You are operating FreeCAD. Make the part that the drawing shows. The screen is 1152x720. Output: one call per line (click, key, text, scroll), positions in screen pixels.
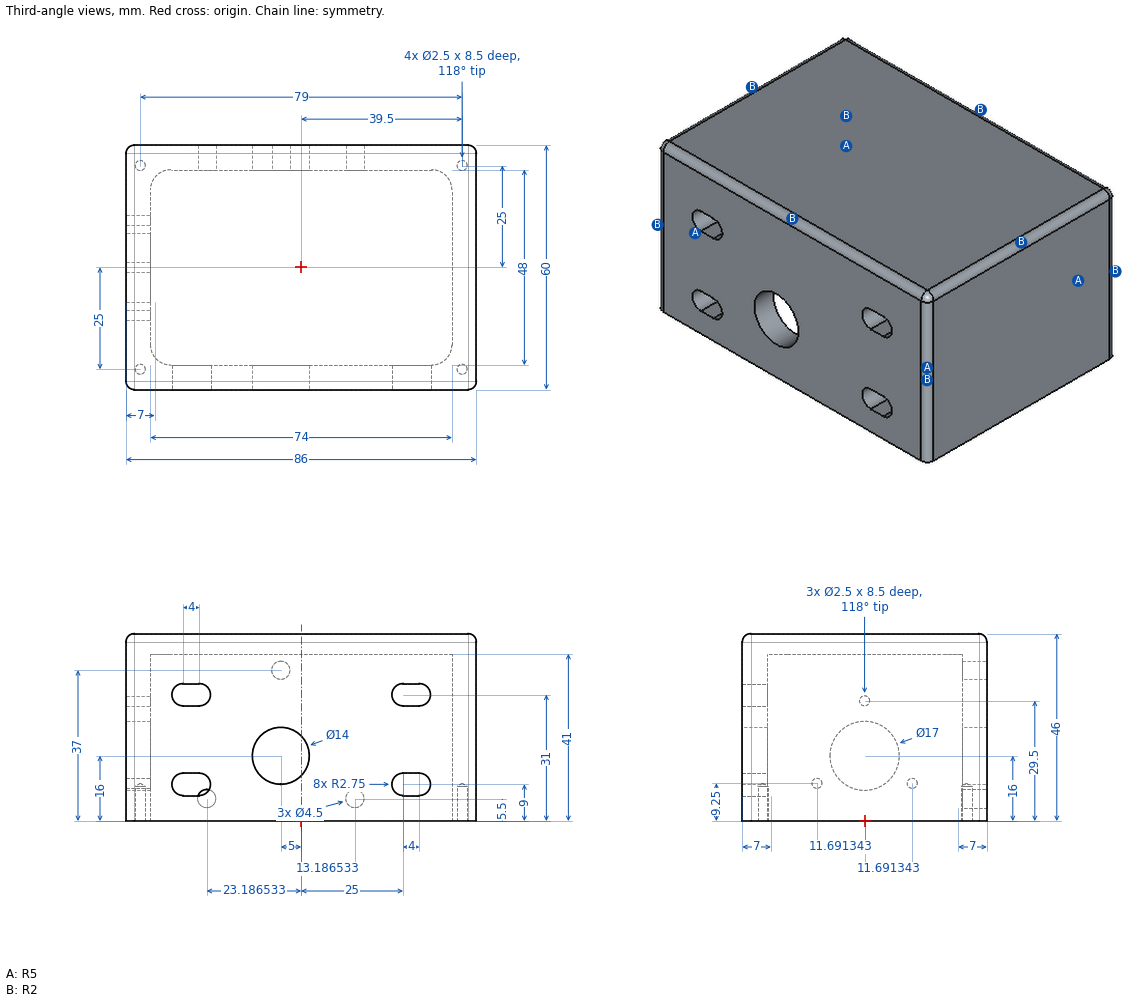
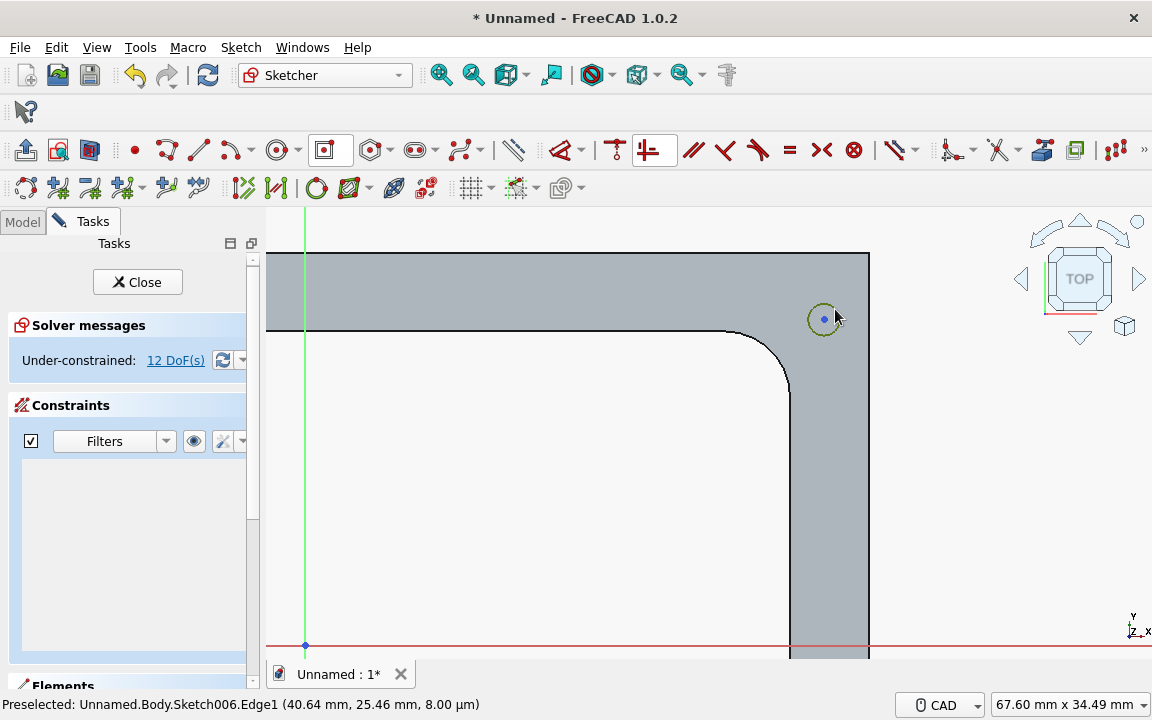
scroll(836, 309, down, 5)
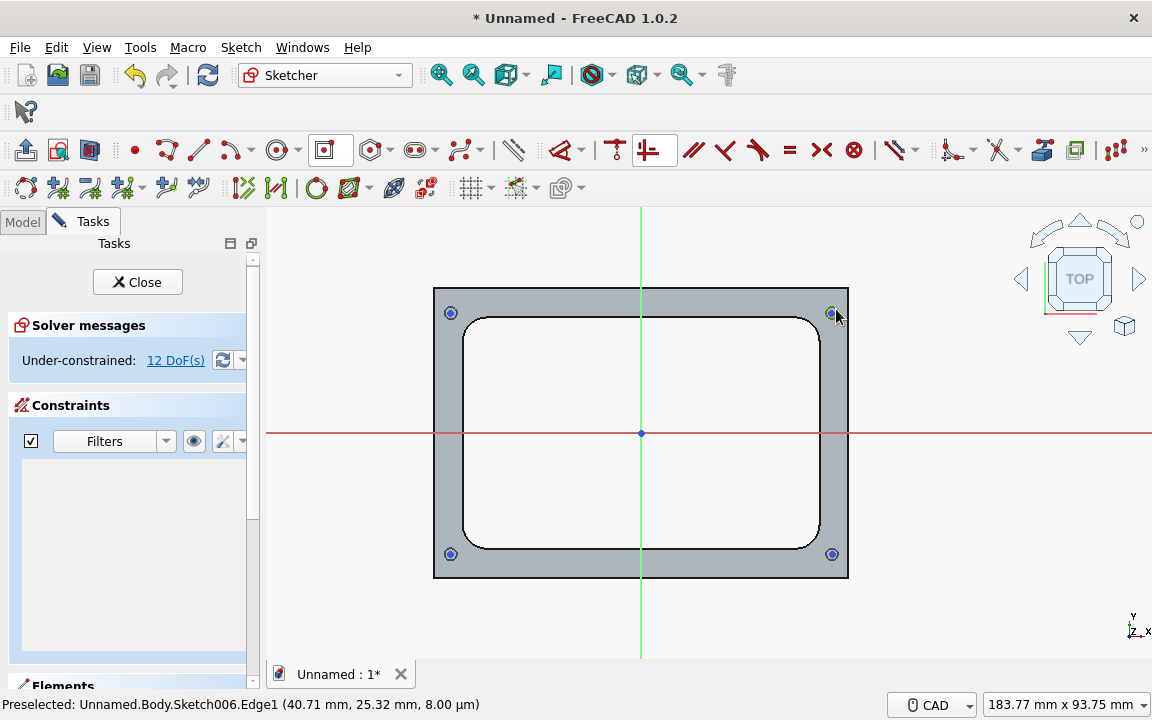
scroll(455, 309, up, 5)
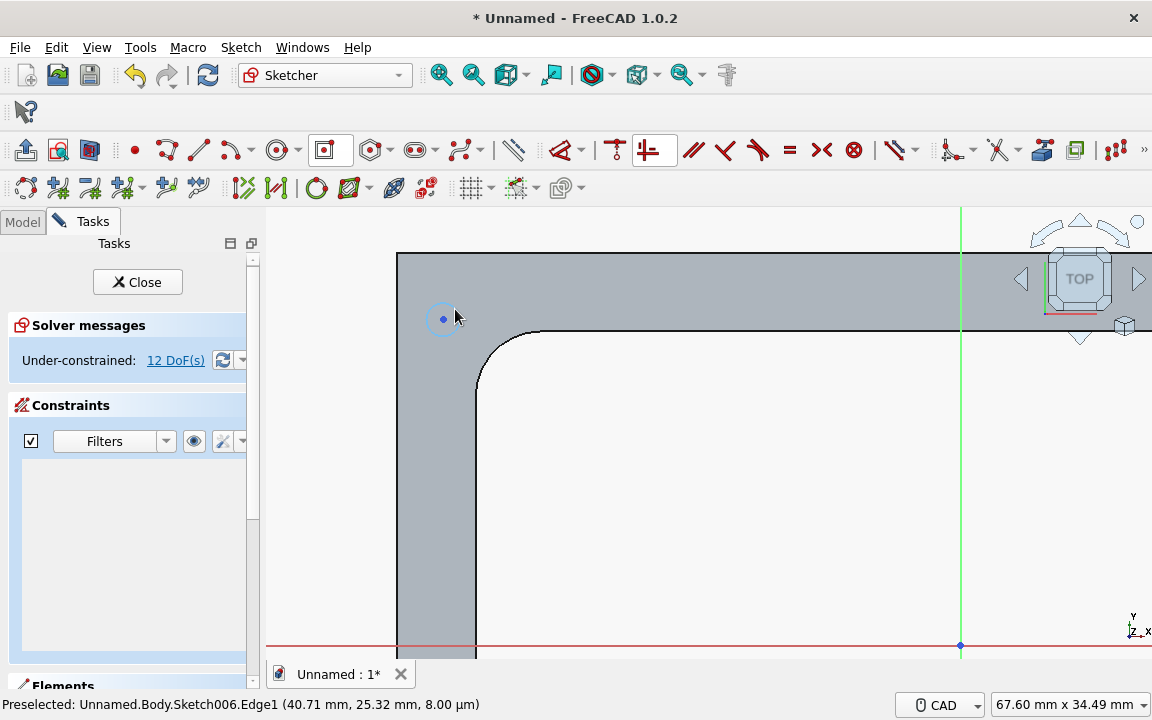
click(455, 308)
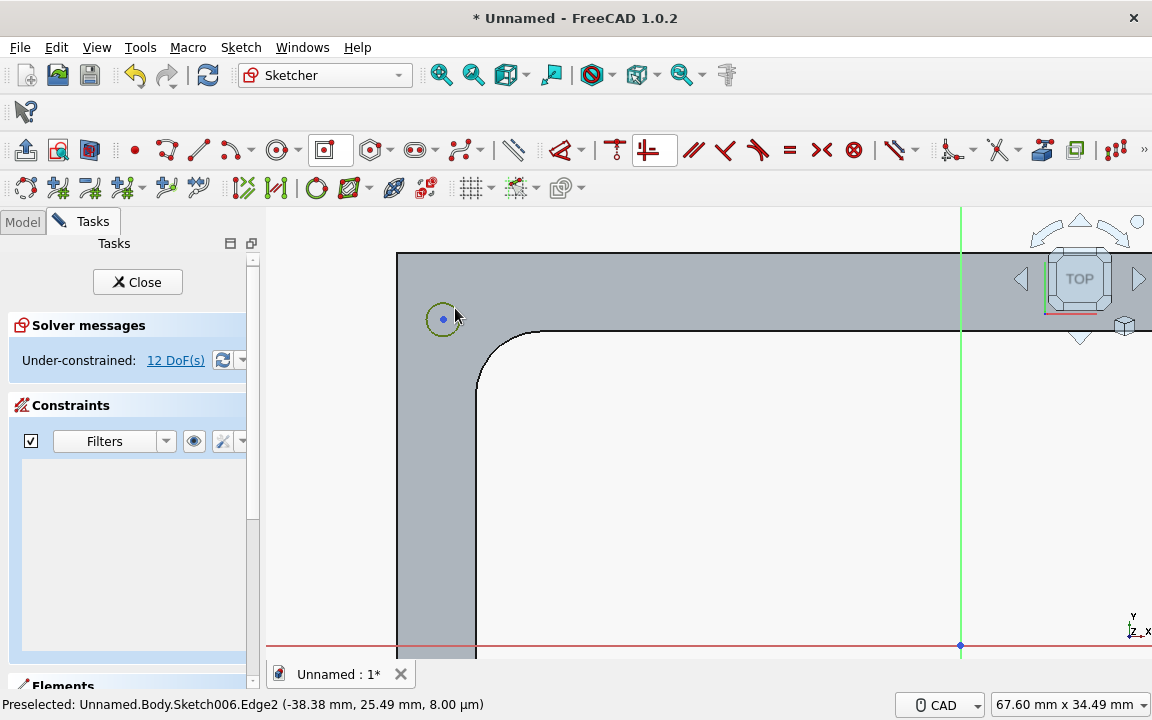
scroll(454, 309, down, 5)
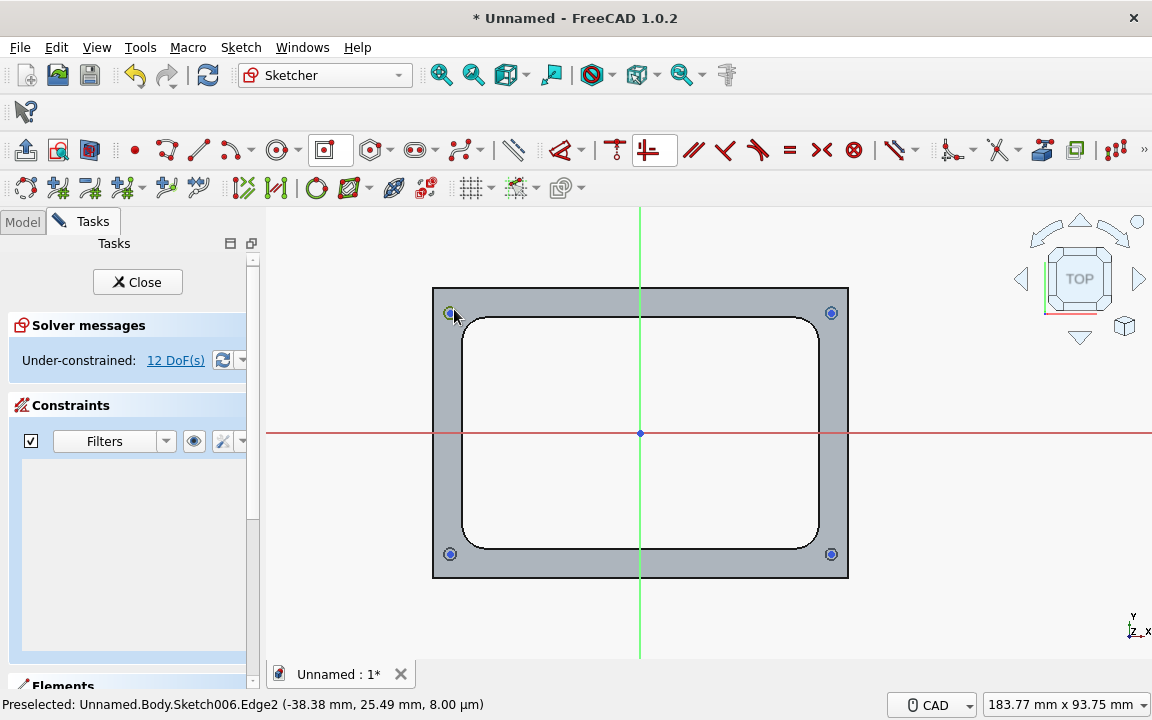
scroll(454, 550, up, 5)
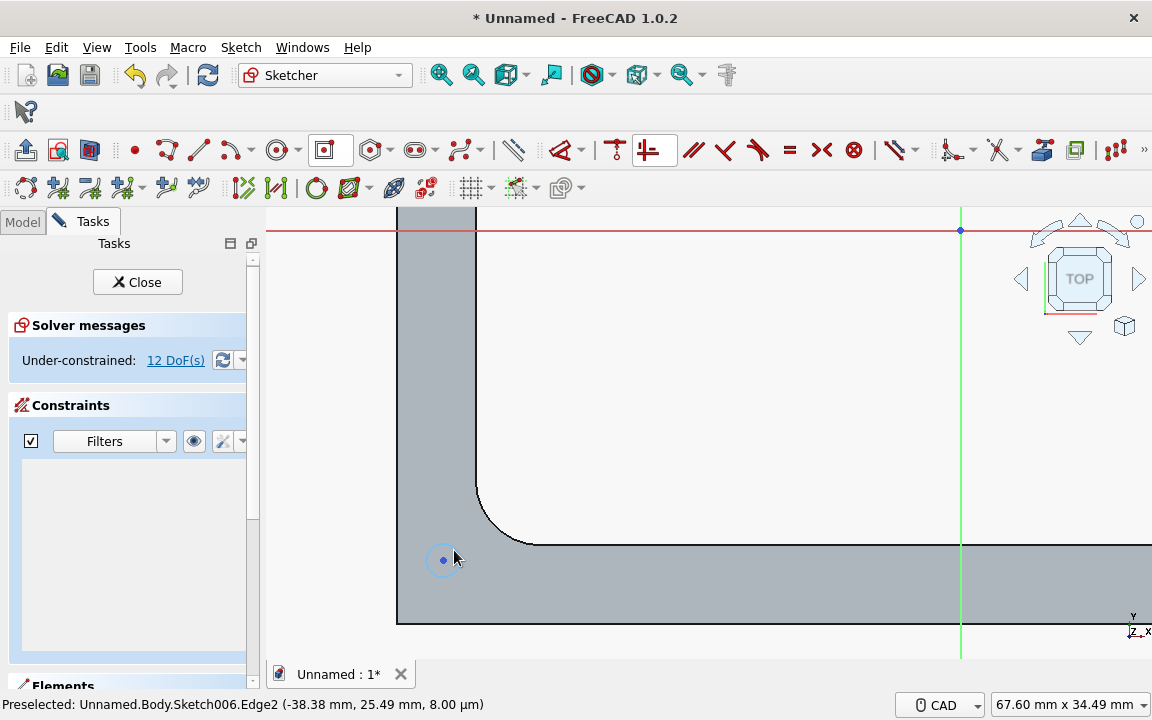
click(455, 549)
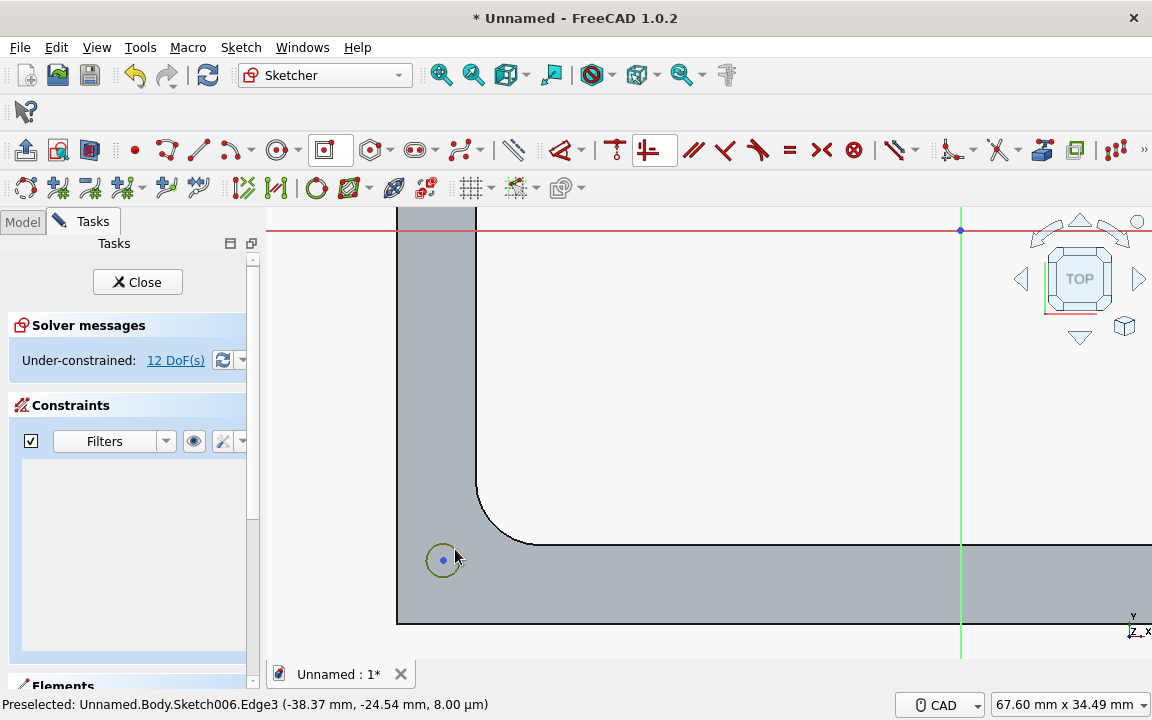
scroll(454, 551, down, 5)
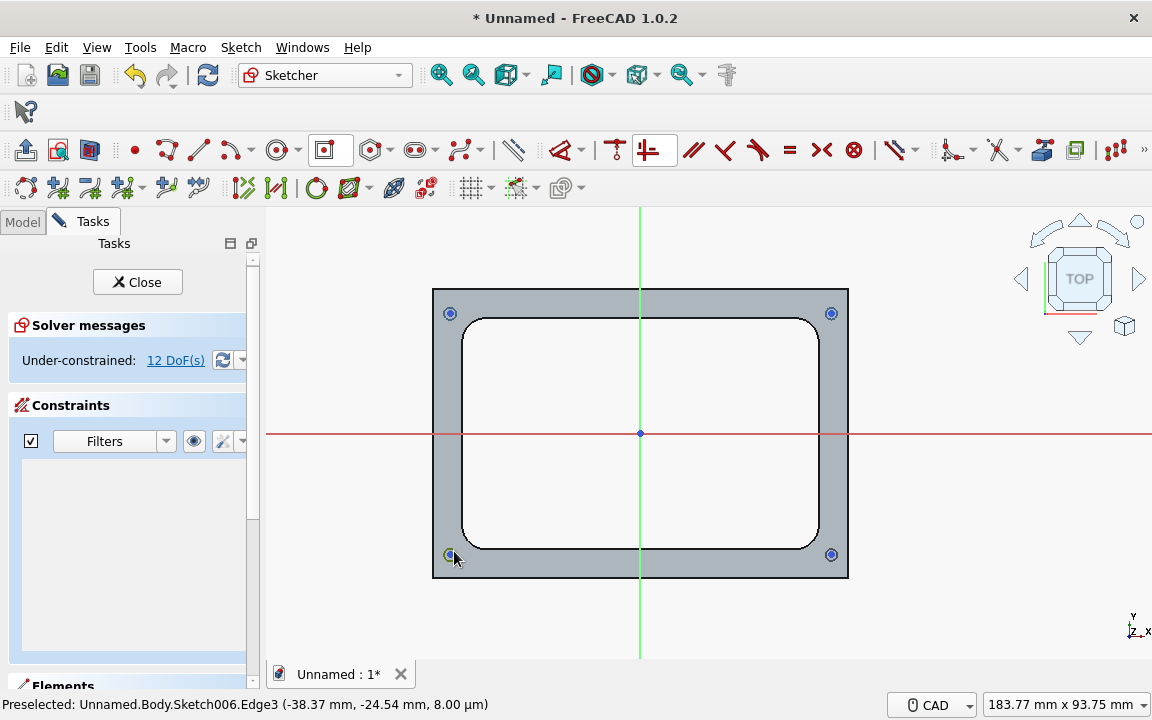
scroll(835, 551, up, 5)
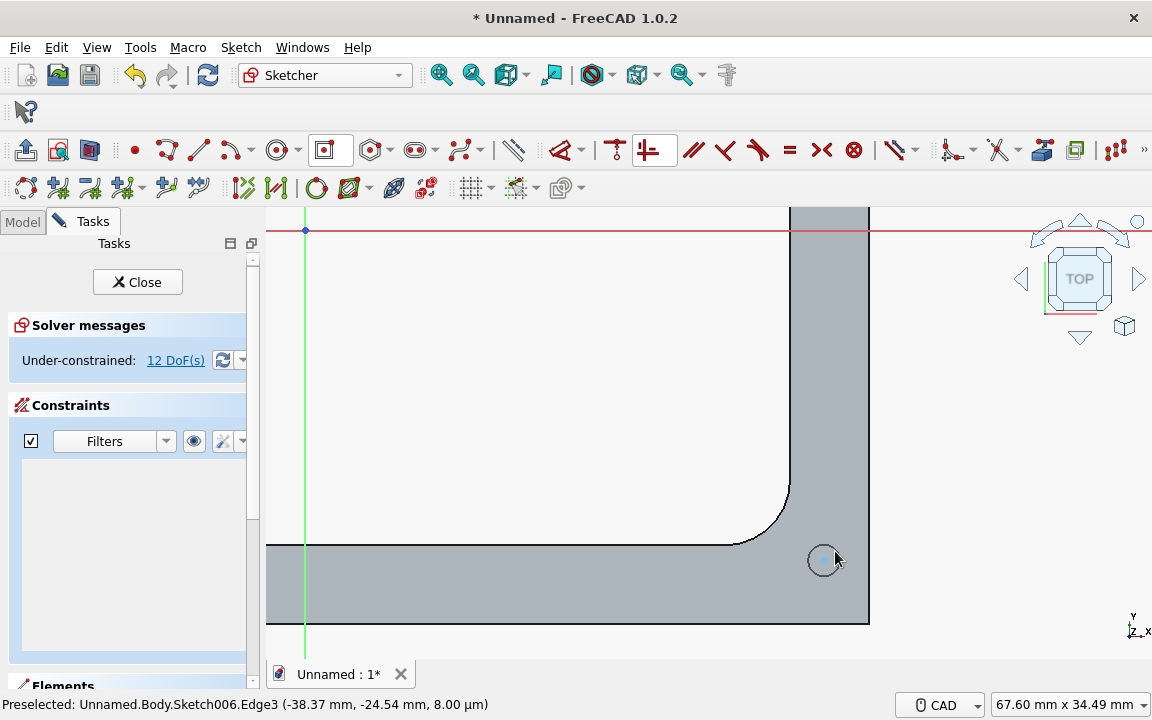
click(835, 549)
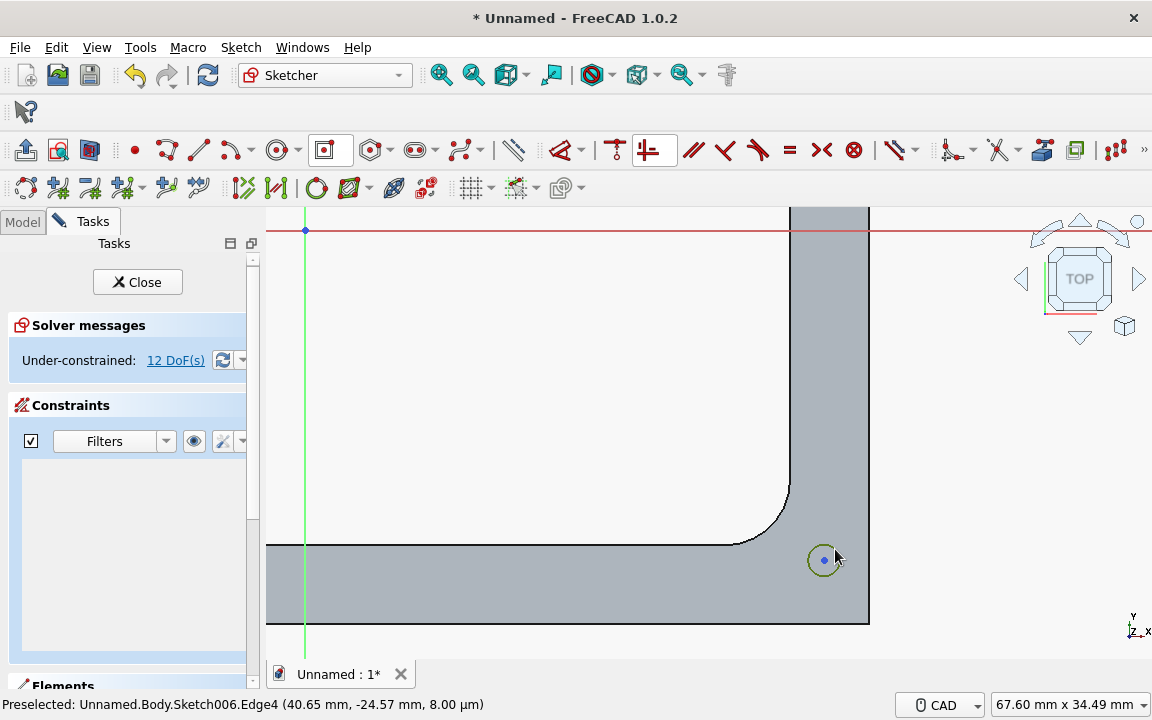
click(790, 150)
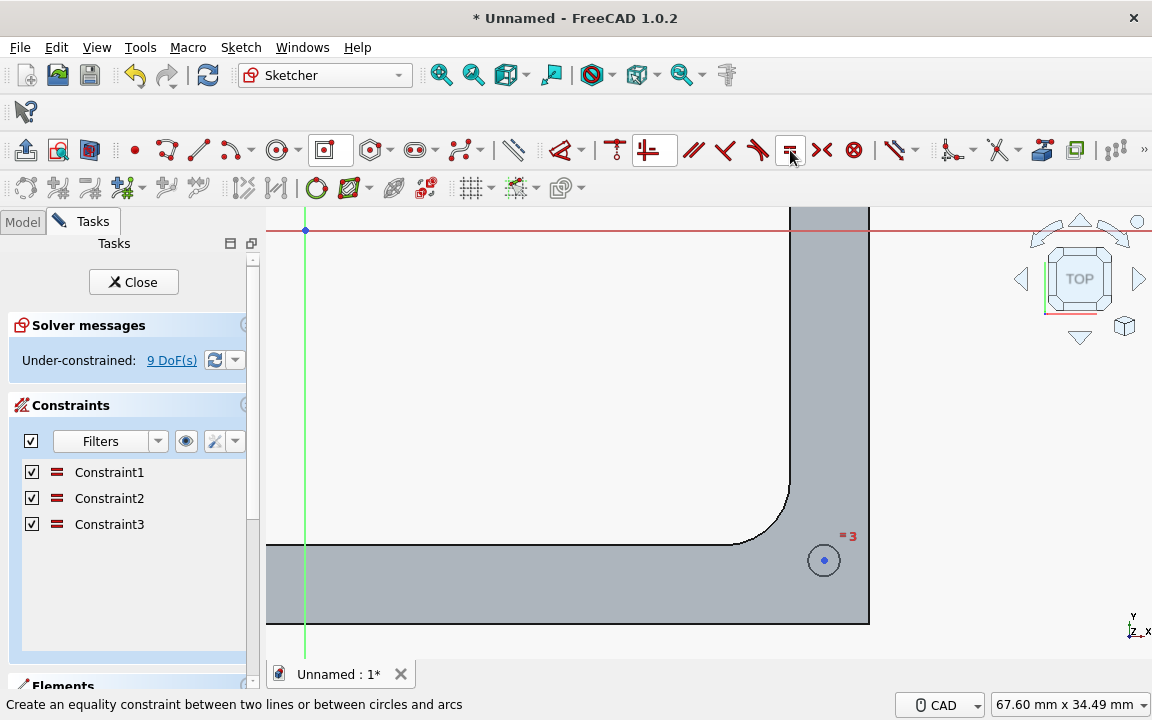
scroll(836, 551, down, 5)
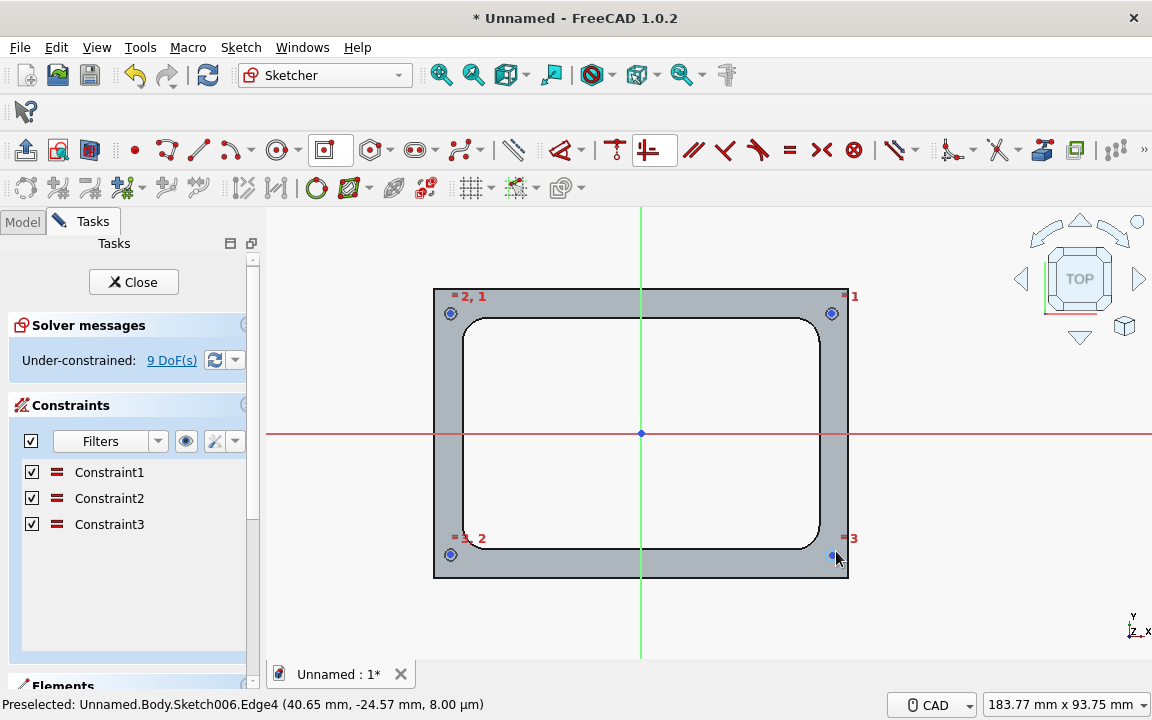
click(832, 314)